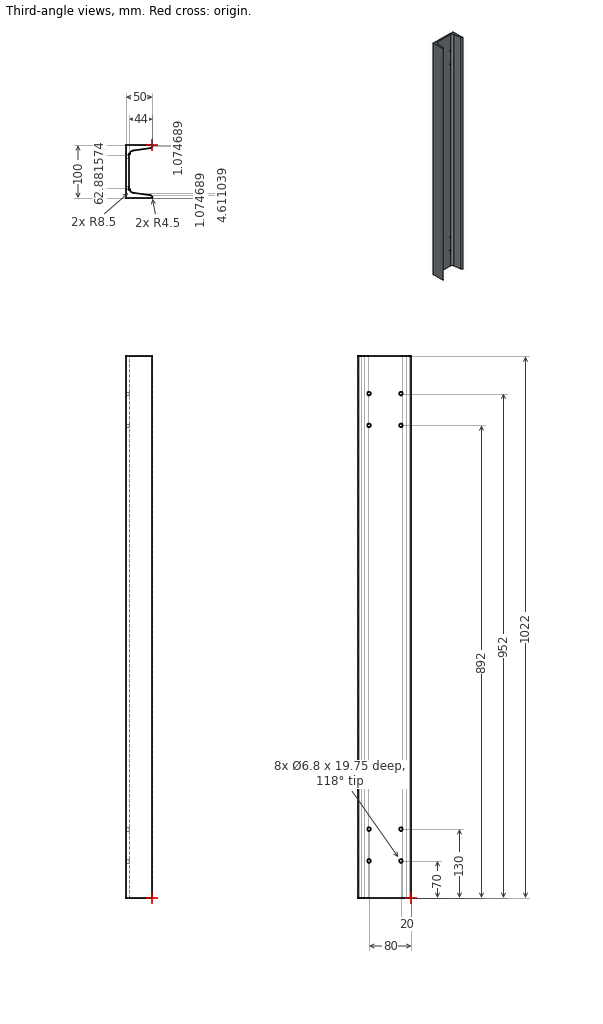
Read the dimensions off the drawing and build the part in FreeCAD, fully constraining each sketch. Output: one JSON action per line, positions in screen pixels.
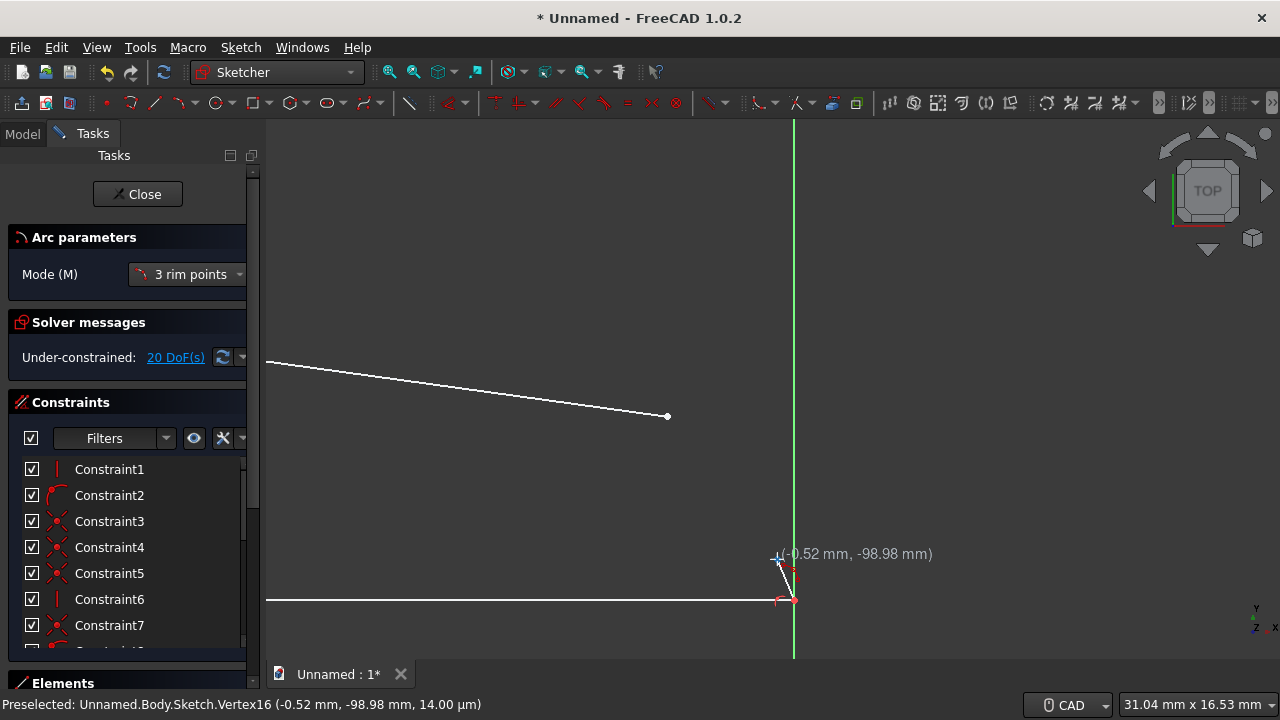
{"action": "scroll", "coordinate": [795, 567], "scroll_direction": "down", "scroll_amount": 11}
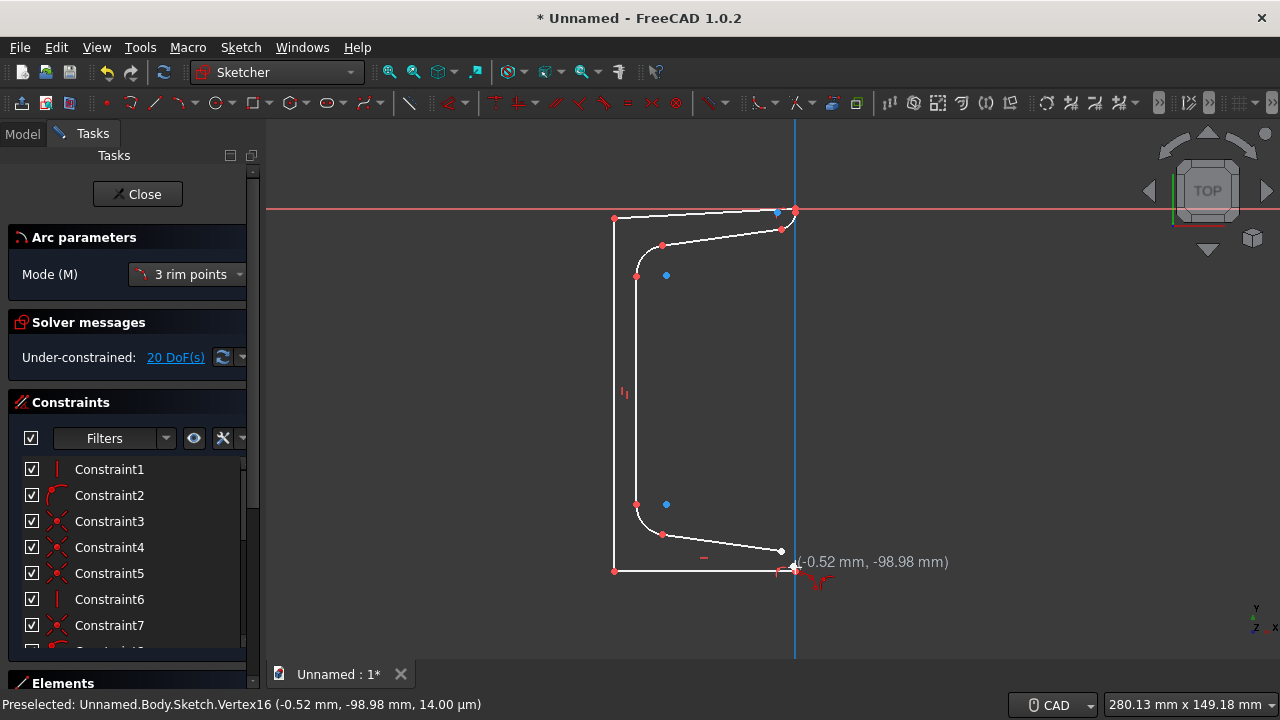
{"action": "left_click", "coordinate": [781, 551]}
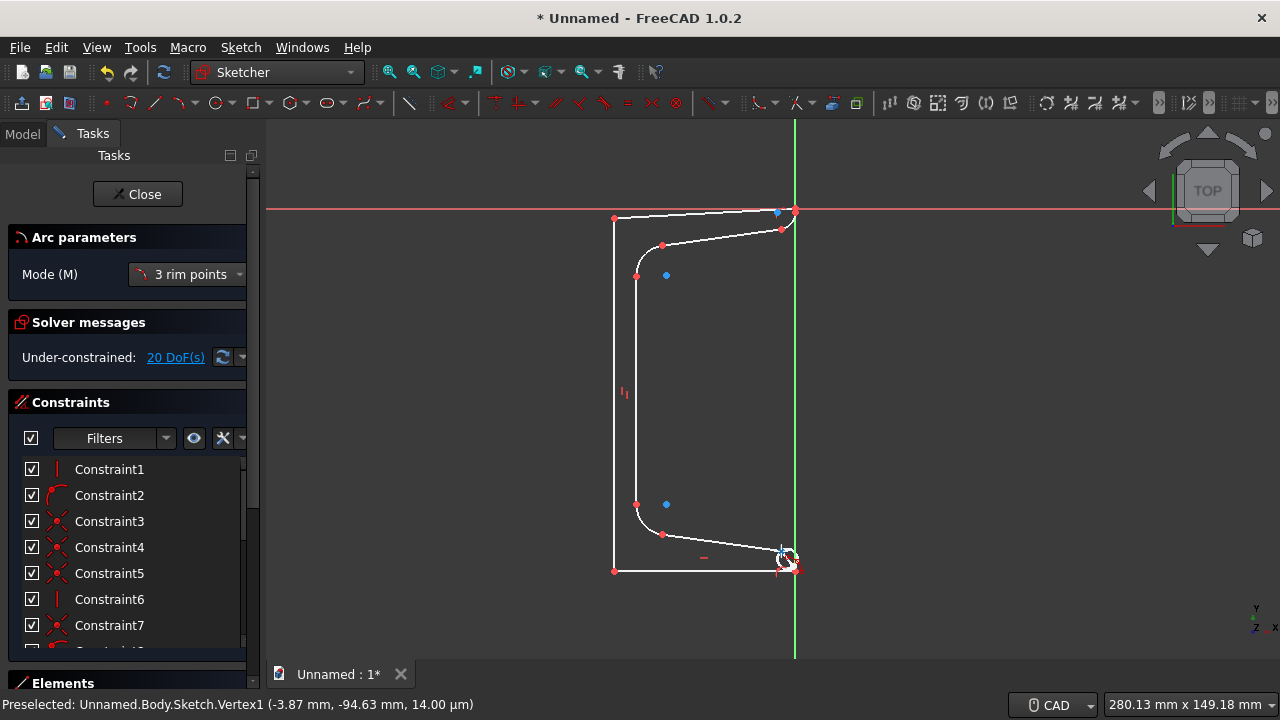
{"action": "scroll", "coordinate": [791, 556], "scroll_direction": "up", "scroll_amount": 7}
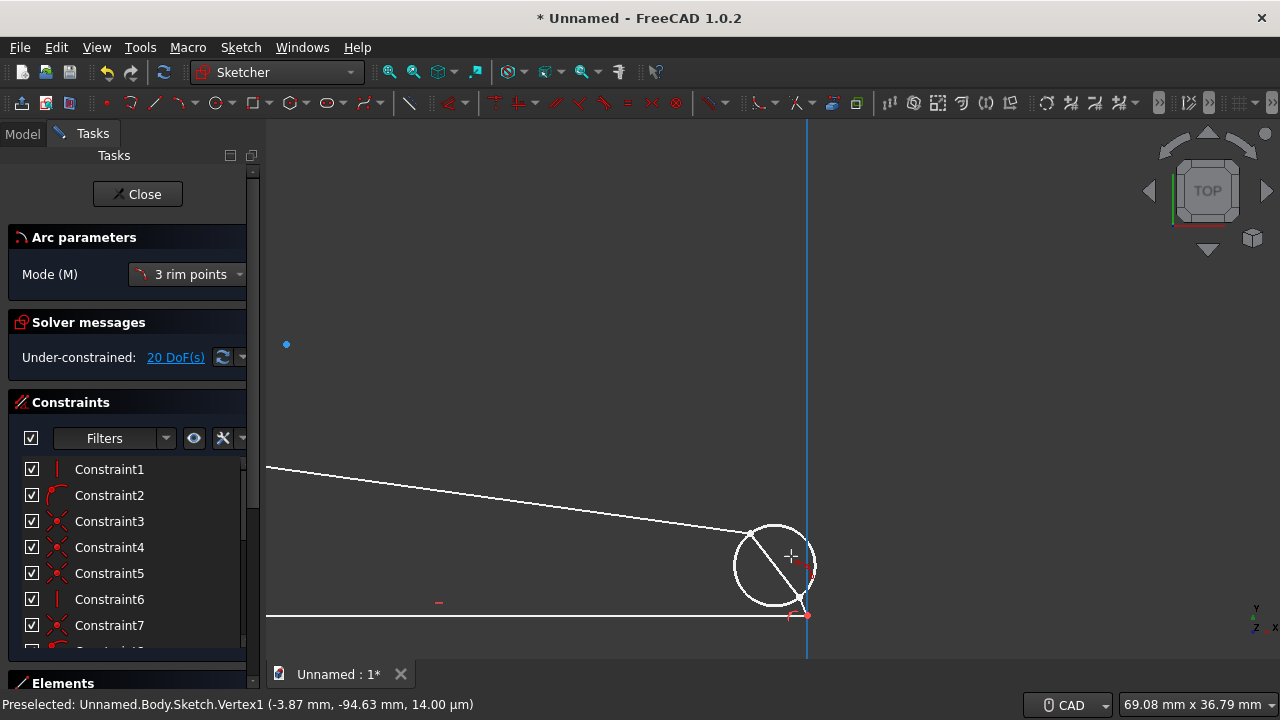
{"action": "left_click", "coordinate": [791, 553]}
{"action": "key", "text": "Escape"}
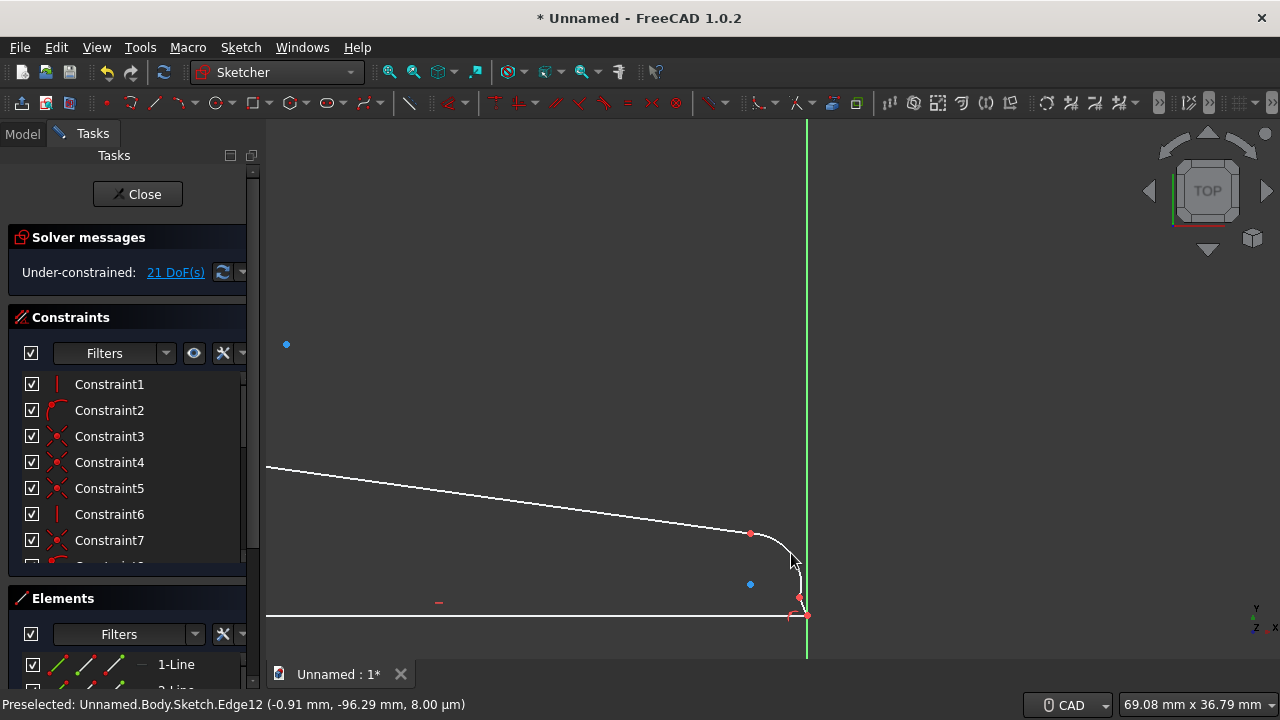
{"action": "scroll", "coordinate": [791, 556], "scroll_direction": "down", "scroll_amount": 7}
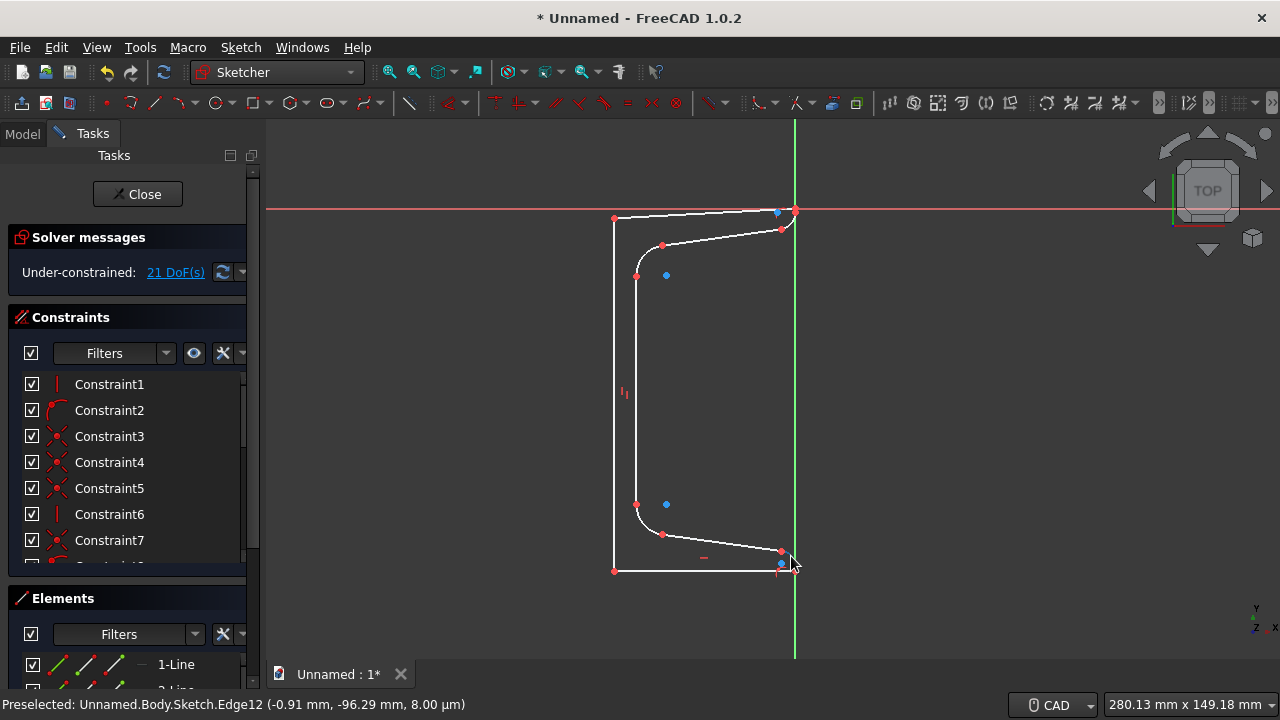
{"action": "left_click", "coordinate": [746, 546]}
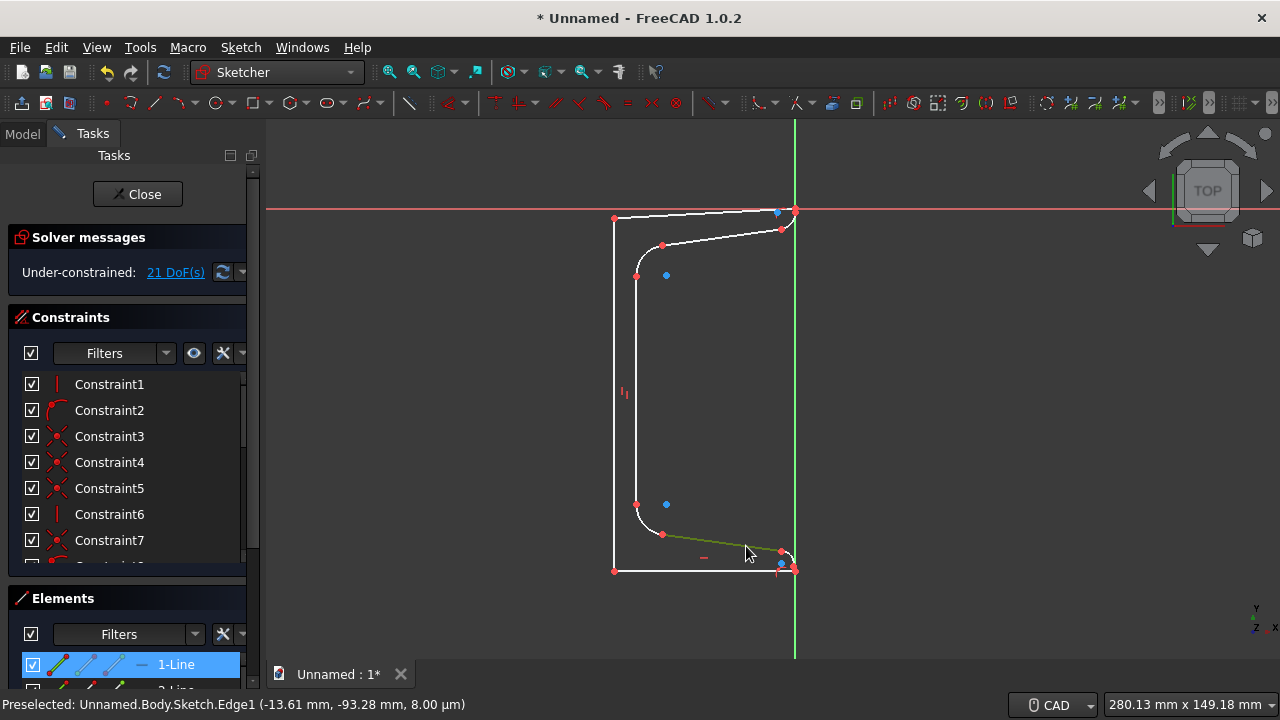
{"action": "left_click", "coordinate": [639, 517]}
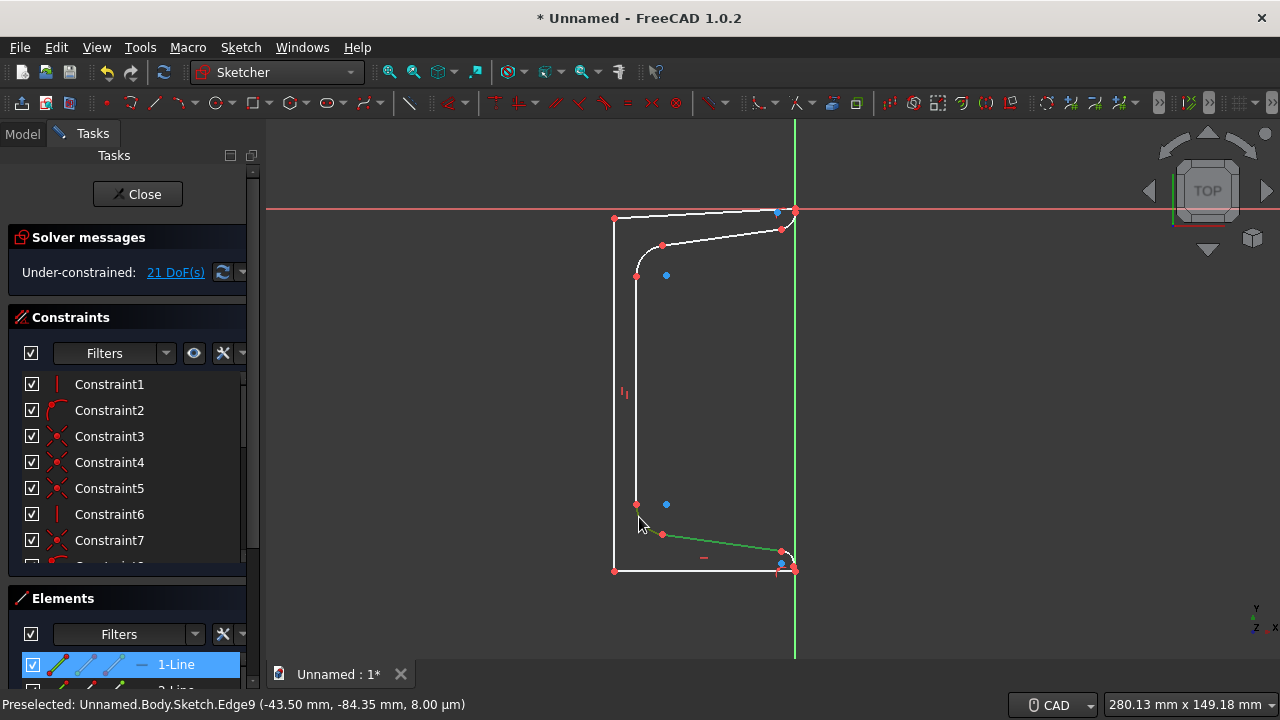
{"action": "left_click", "coordinate": [604, 104]}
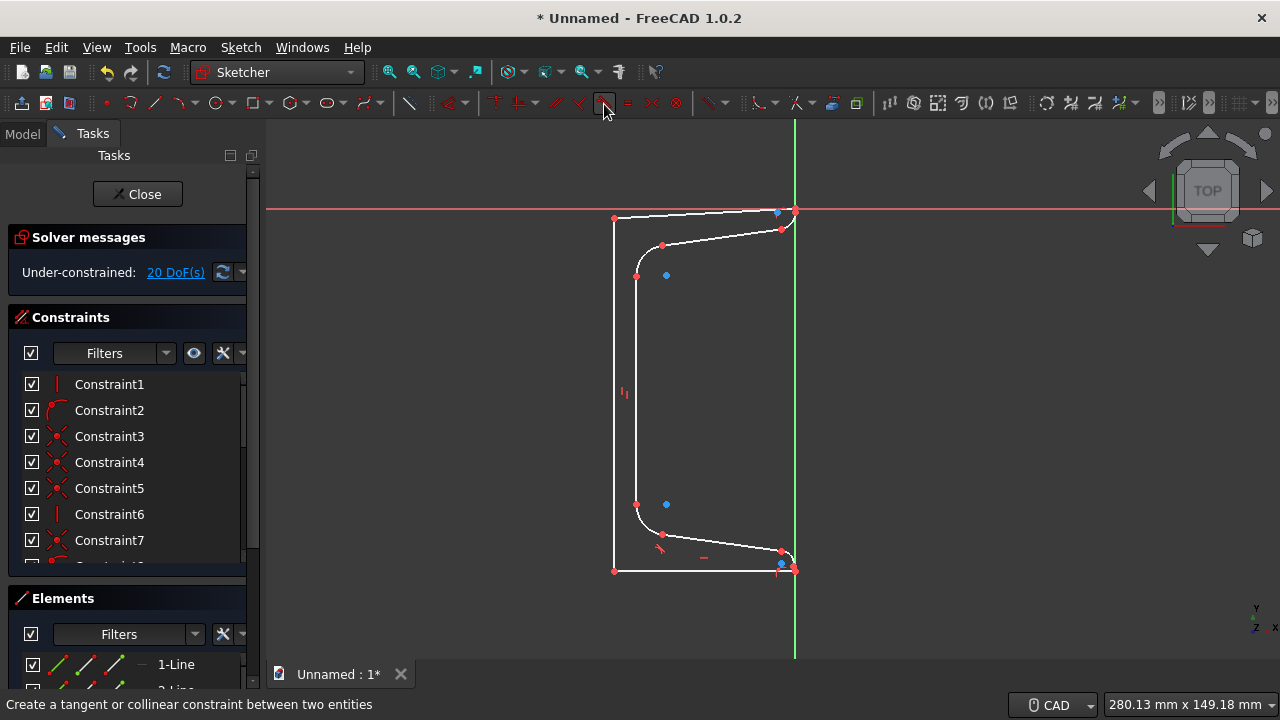
{"action": "left_click", "coordinate": [746, 546]}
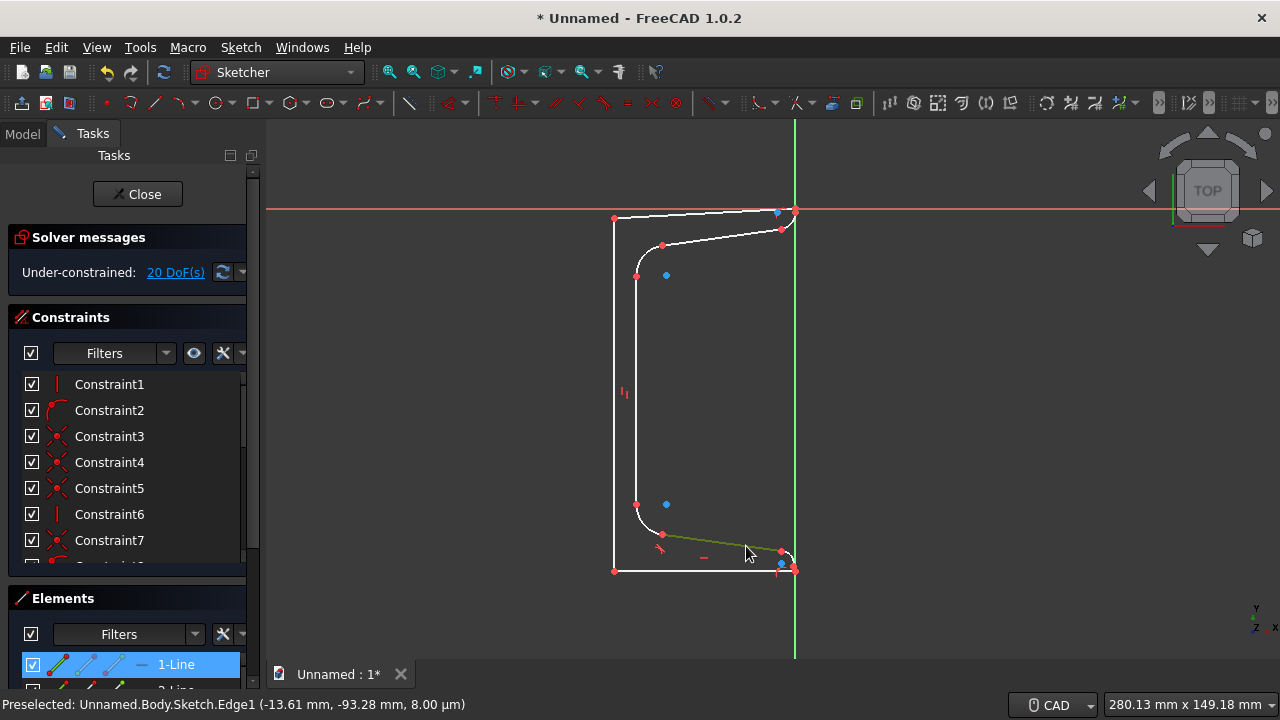
{"action": "scroll", "coordinate": [793, 560], "scroll_direction": "up", "scroll_amount": 4}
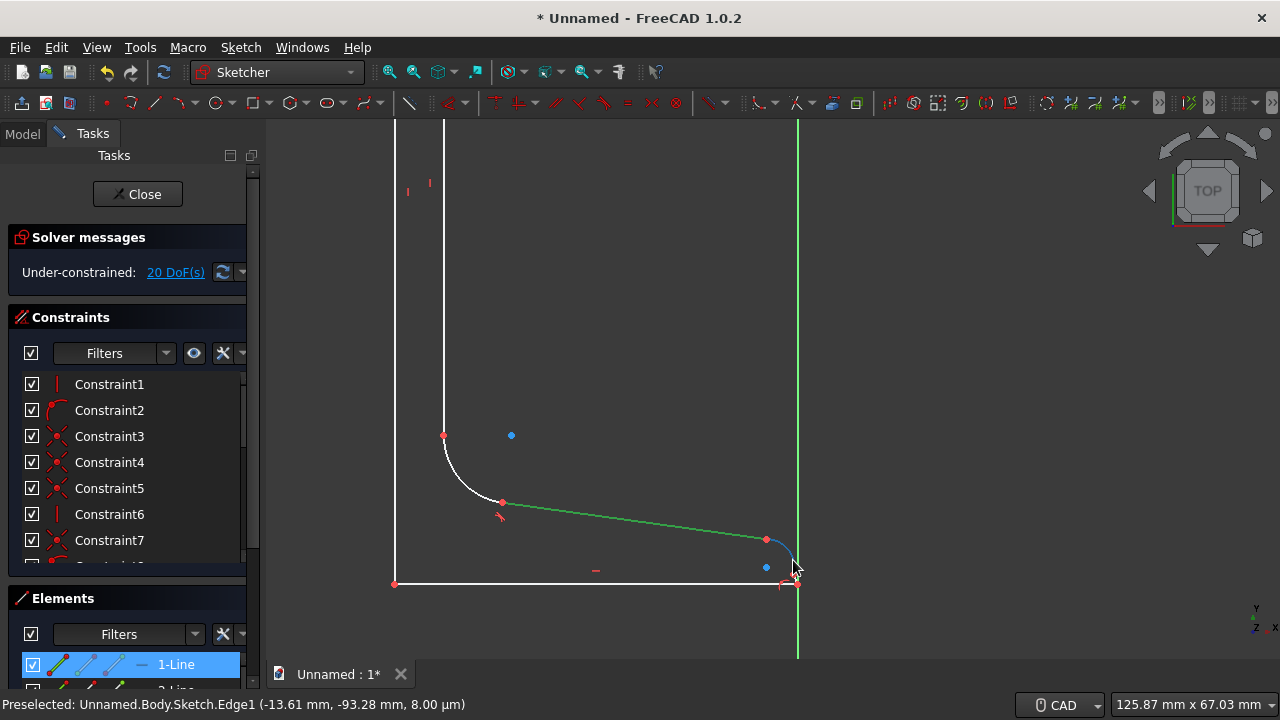
{"action": "left_click", "coordinate": [793, 559]}